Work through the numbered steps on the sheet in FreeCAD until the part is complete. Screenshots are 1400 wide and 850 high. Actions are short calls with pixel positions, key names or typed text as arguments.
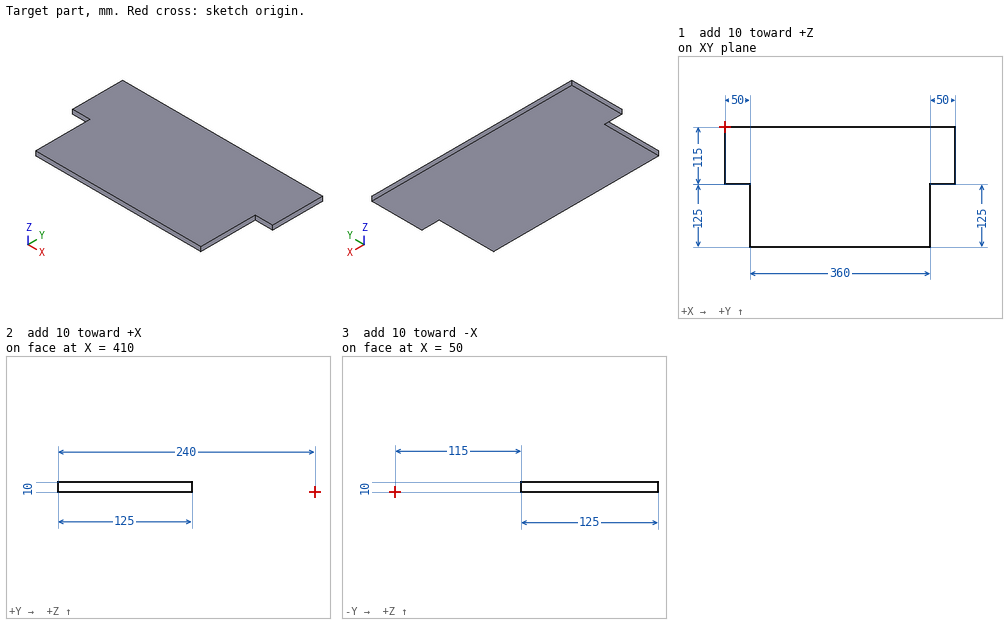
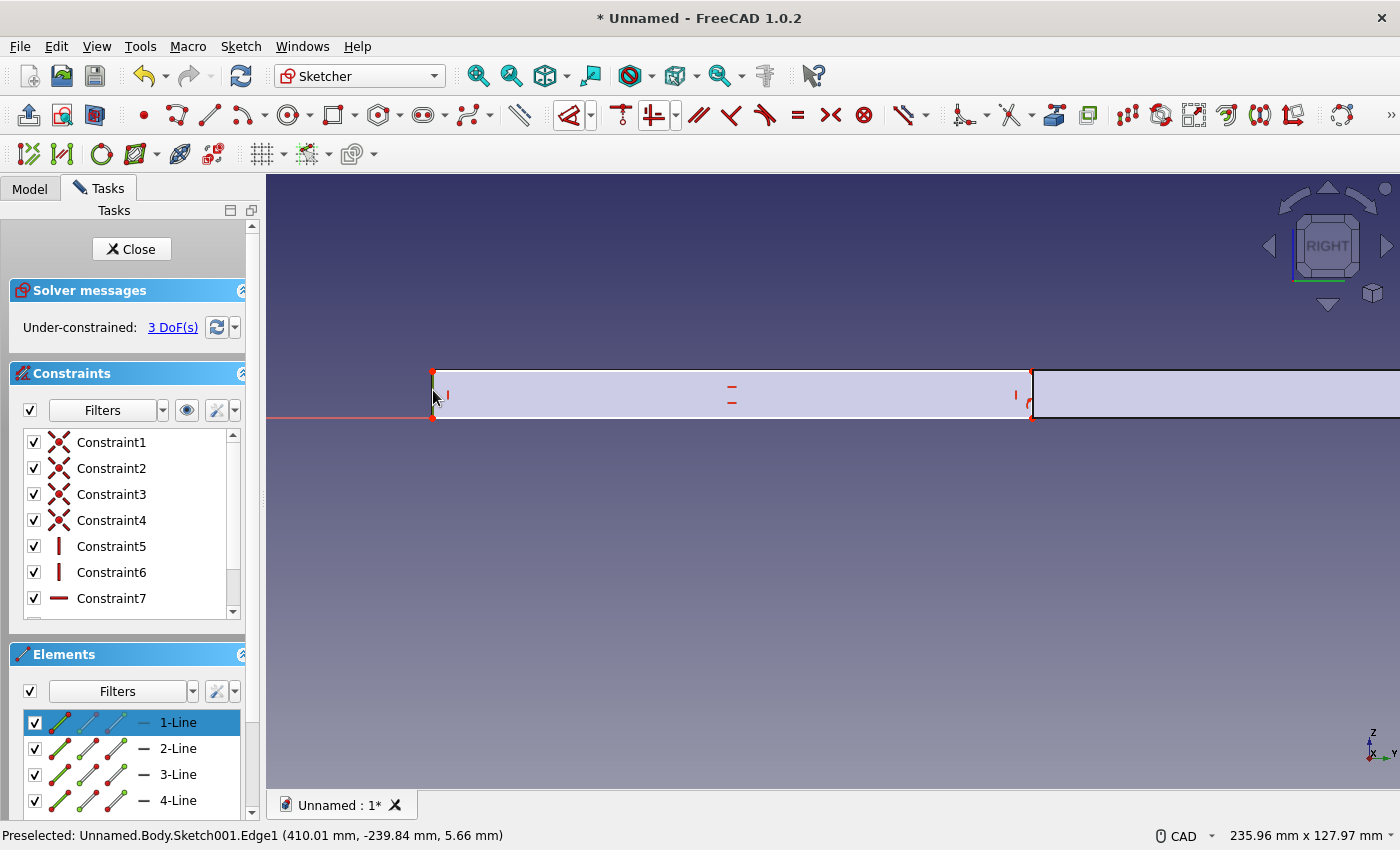
click(590, 116)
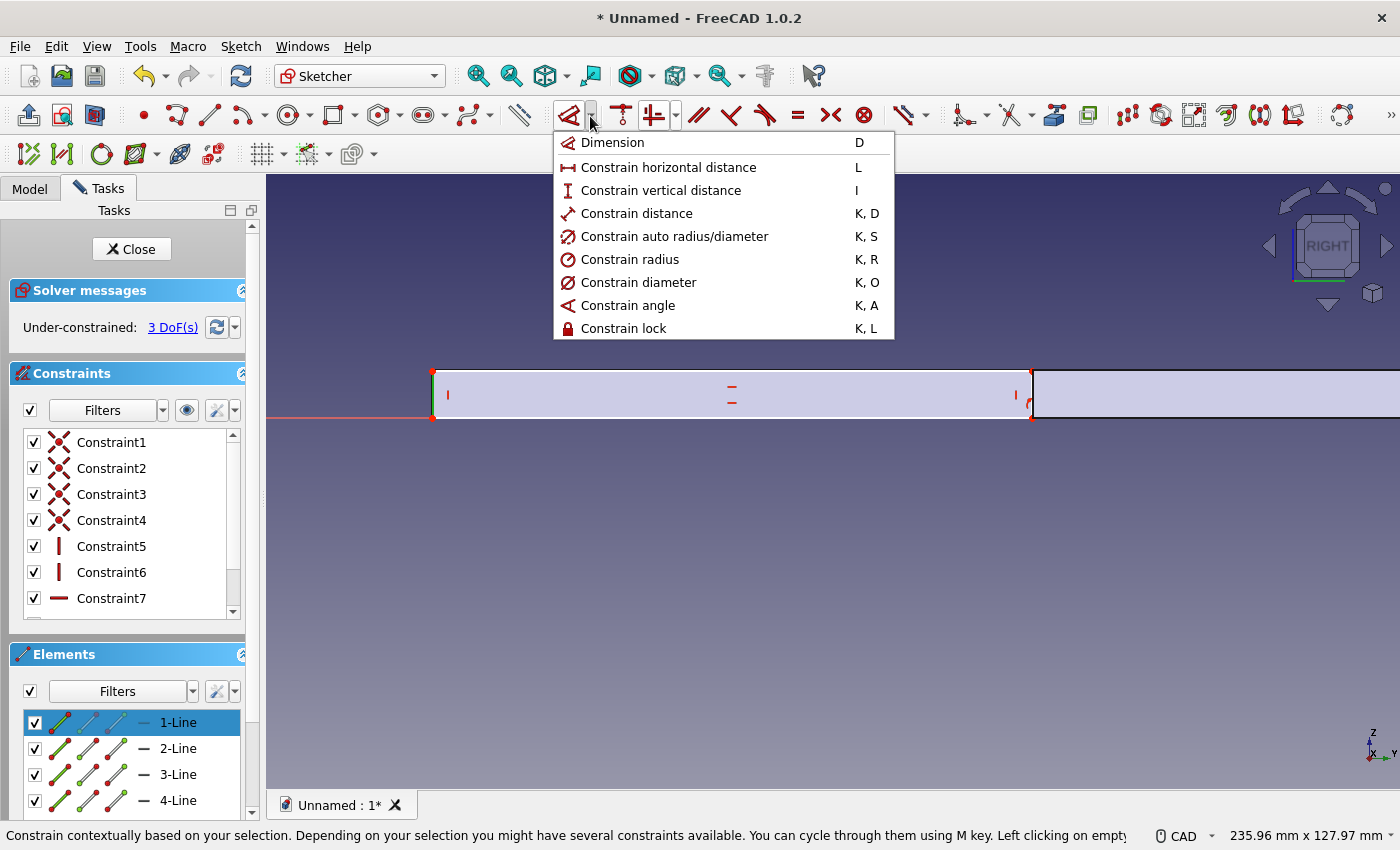
click(724, 190)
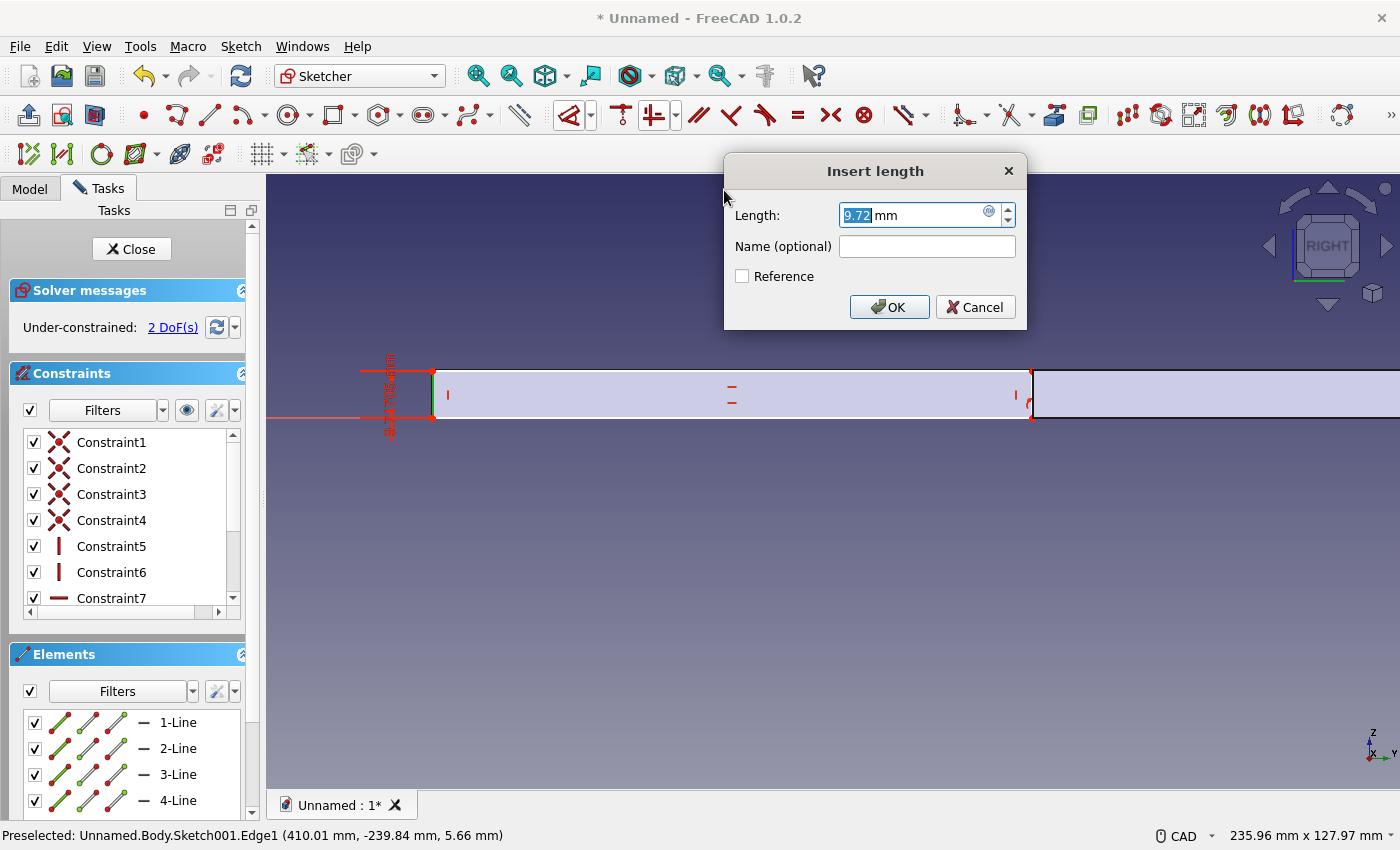
text(10)
key(Return)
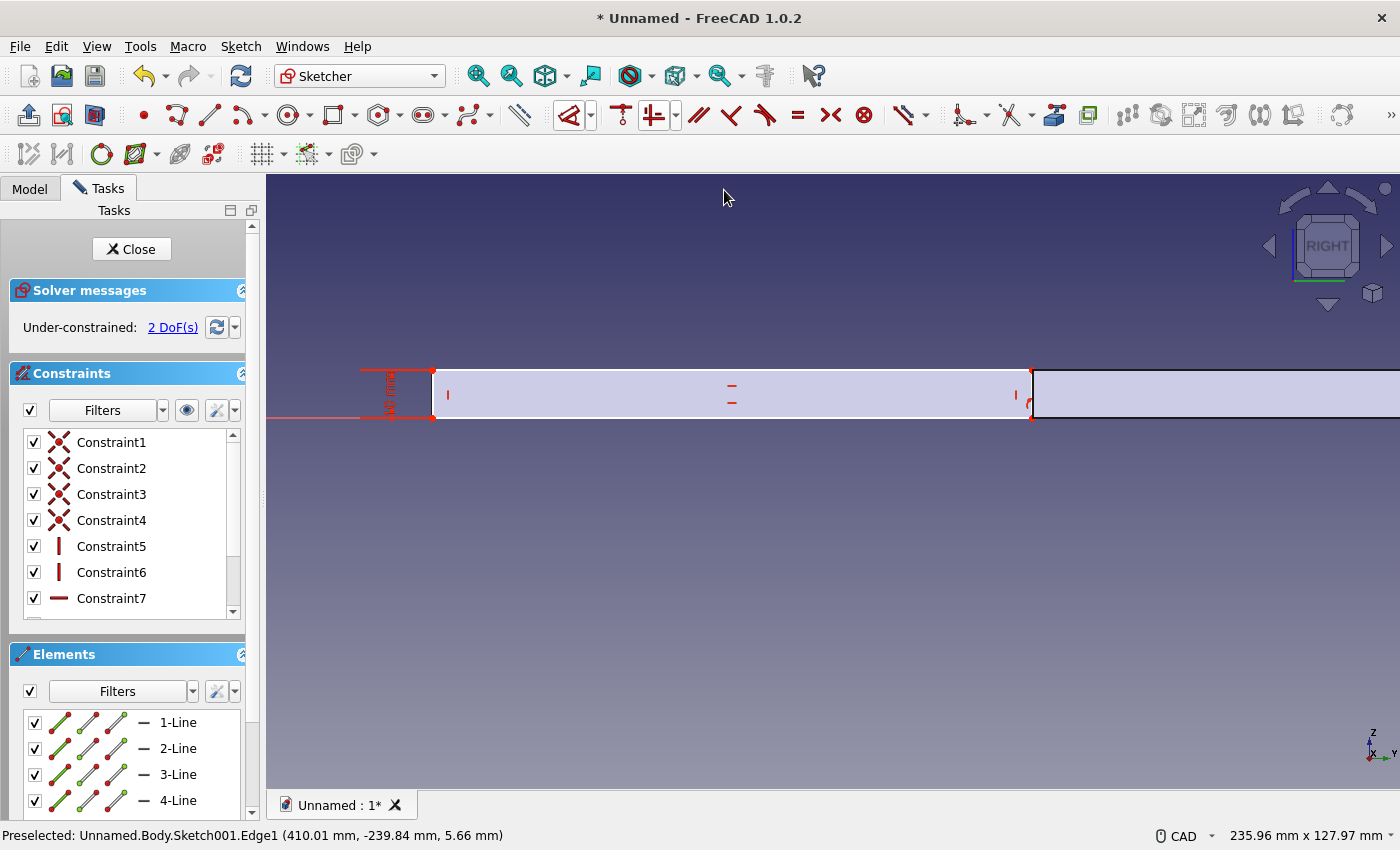
click(613, 418)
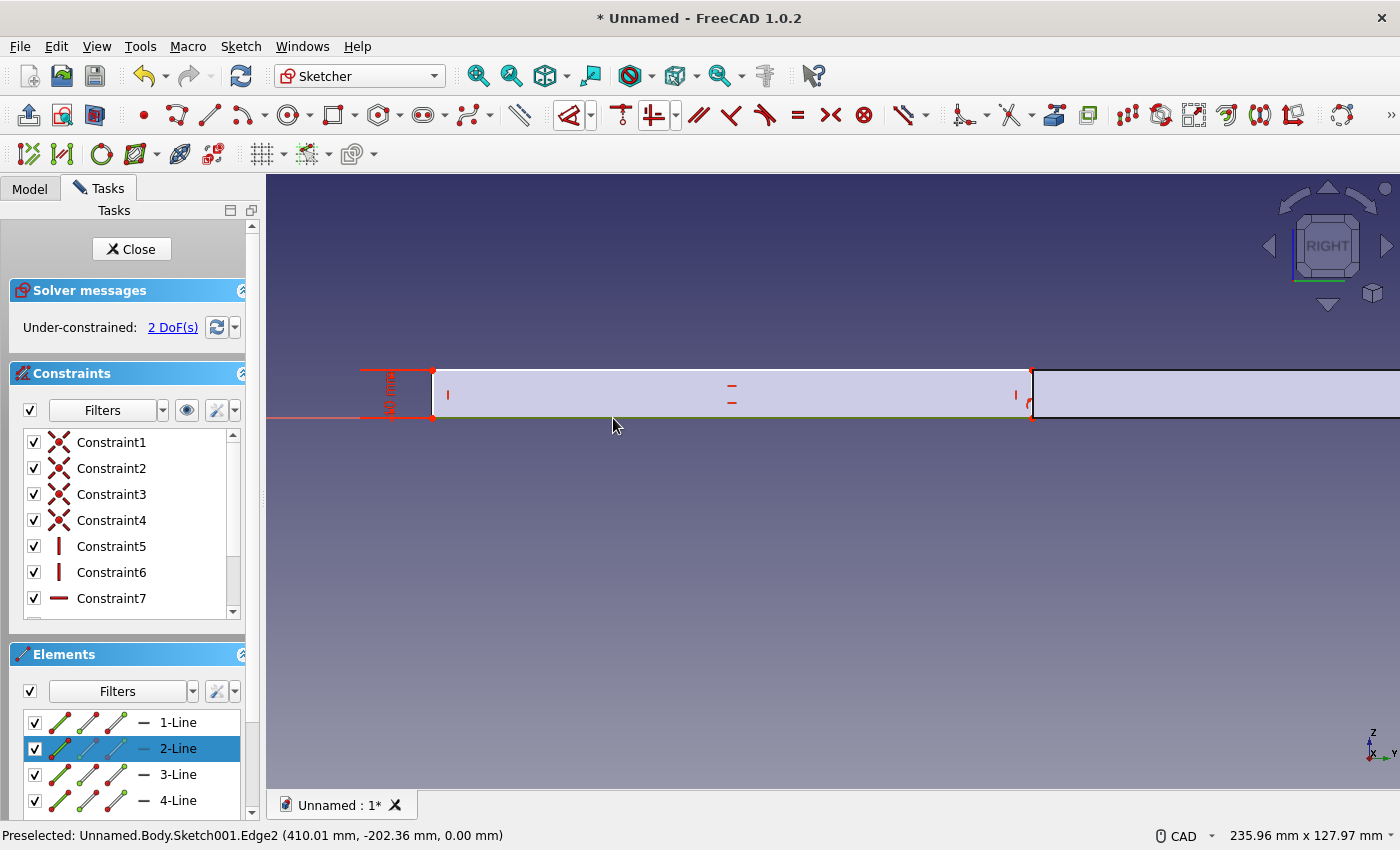
key(l)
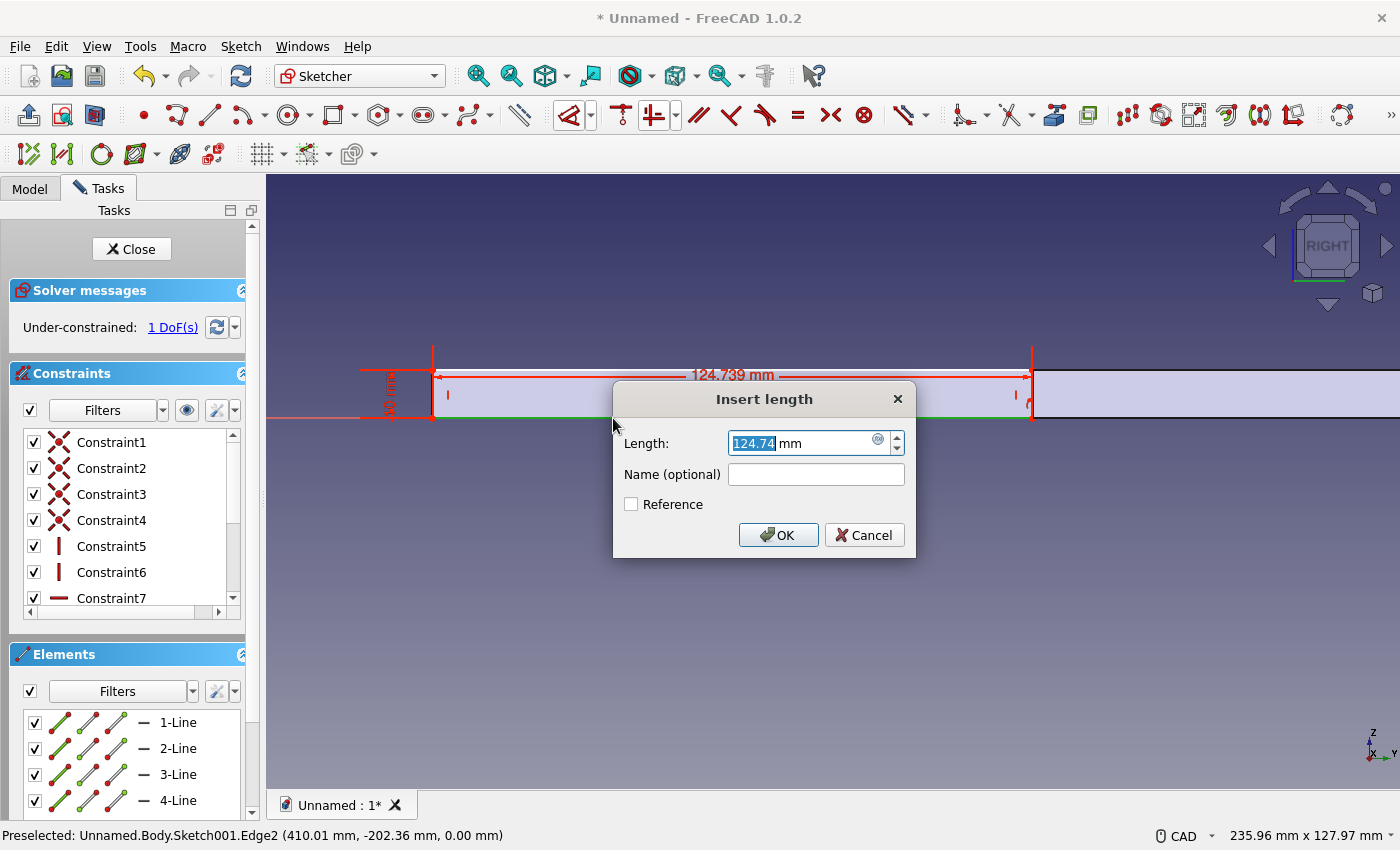
text(125)
key(Return)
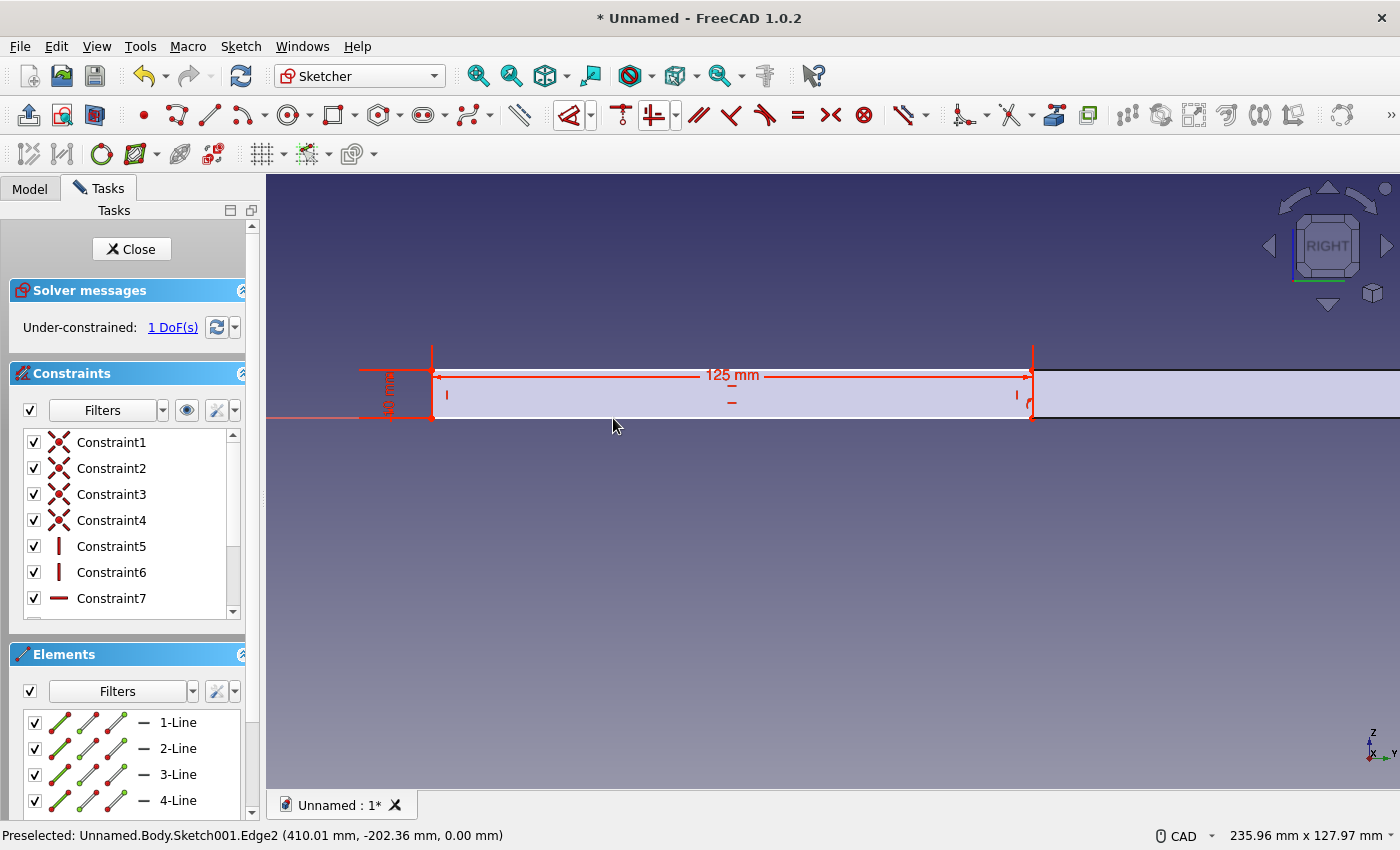
click(432, 370)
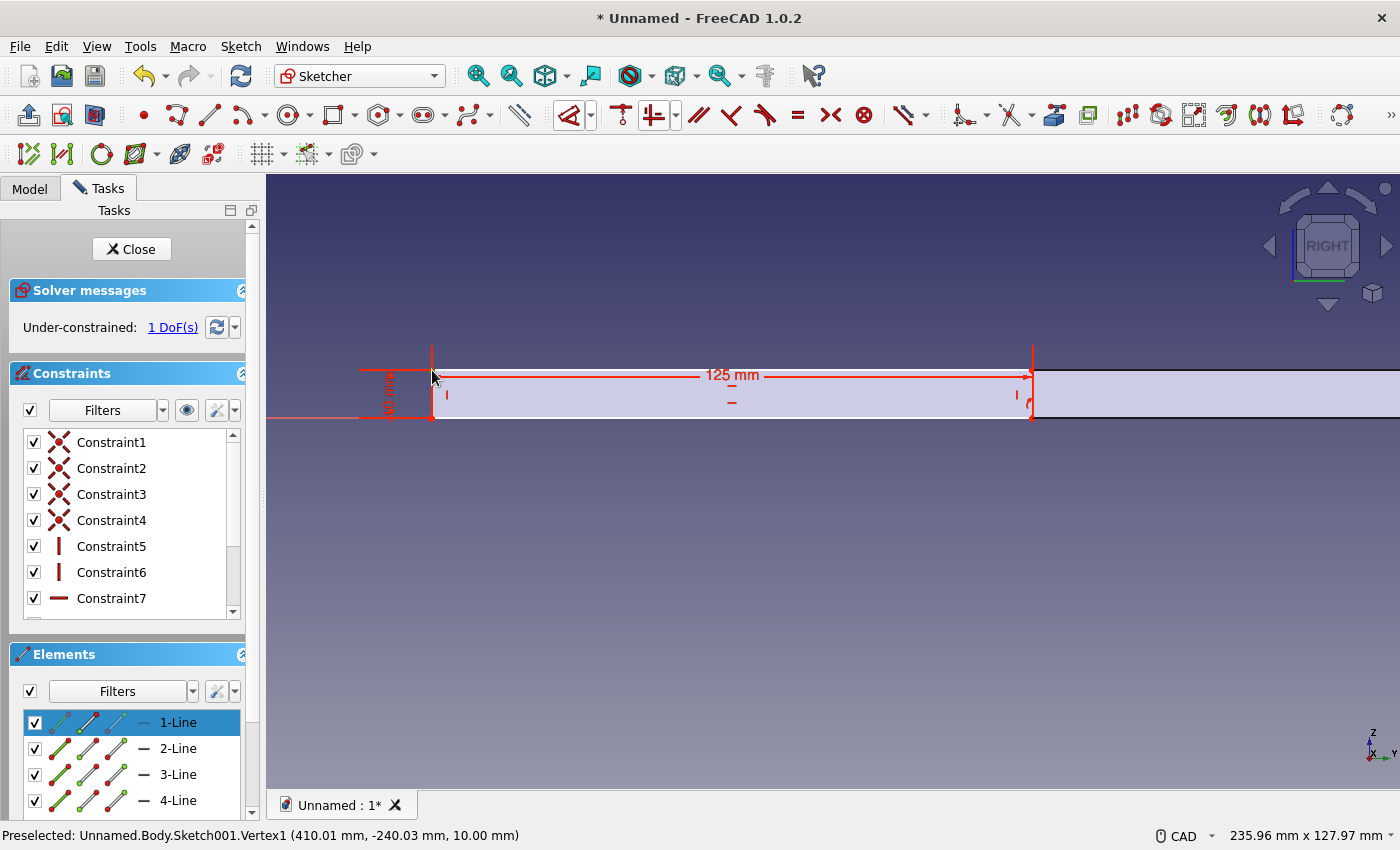
click(590, 116)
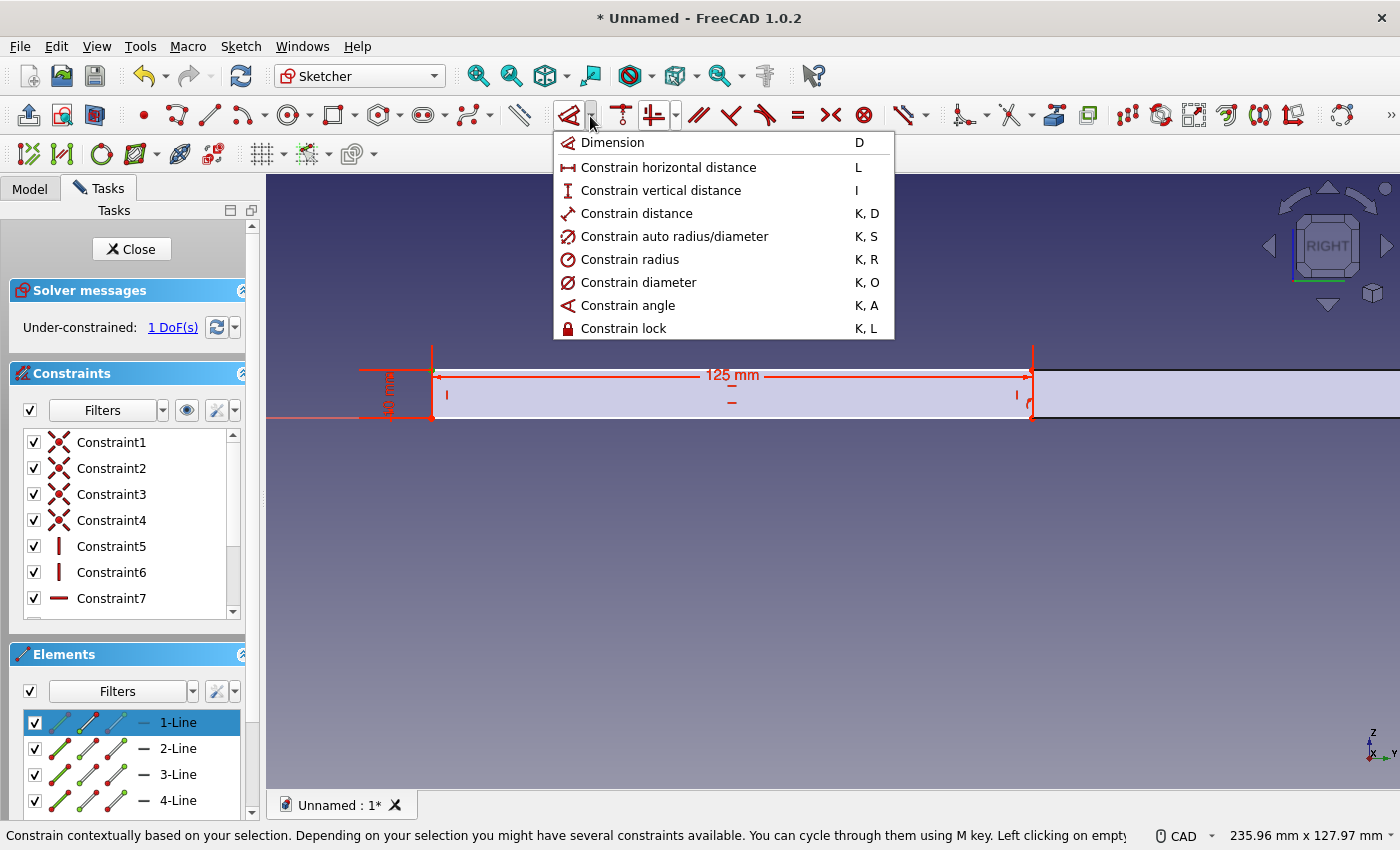
click(724, 168)